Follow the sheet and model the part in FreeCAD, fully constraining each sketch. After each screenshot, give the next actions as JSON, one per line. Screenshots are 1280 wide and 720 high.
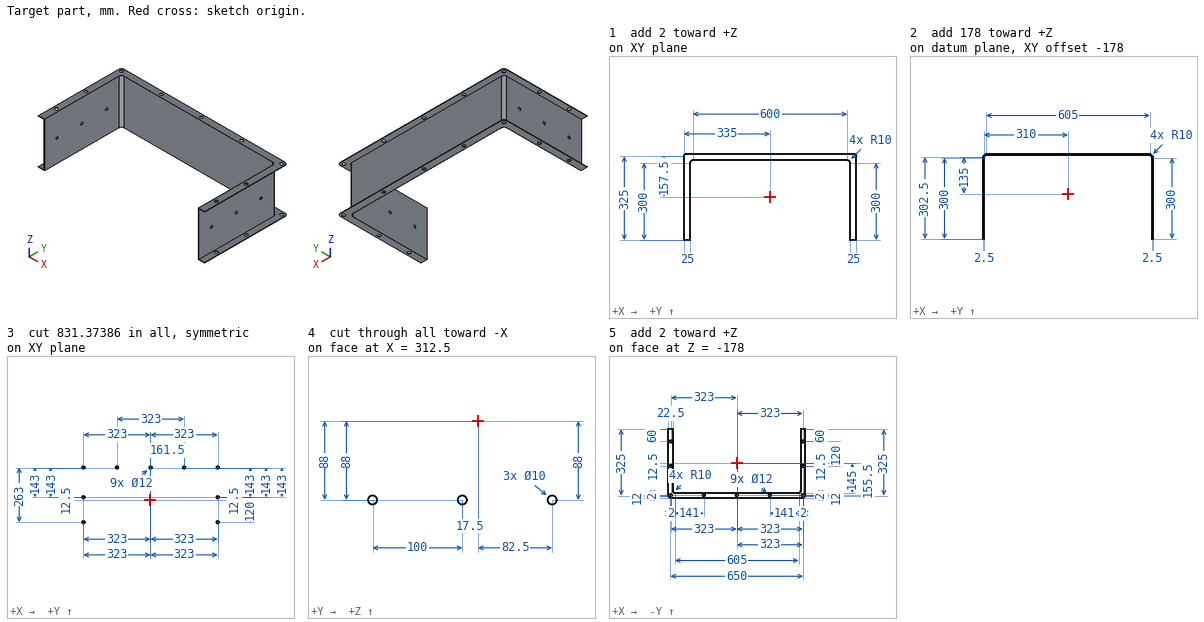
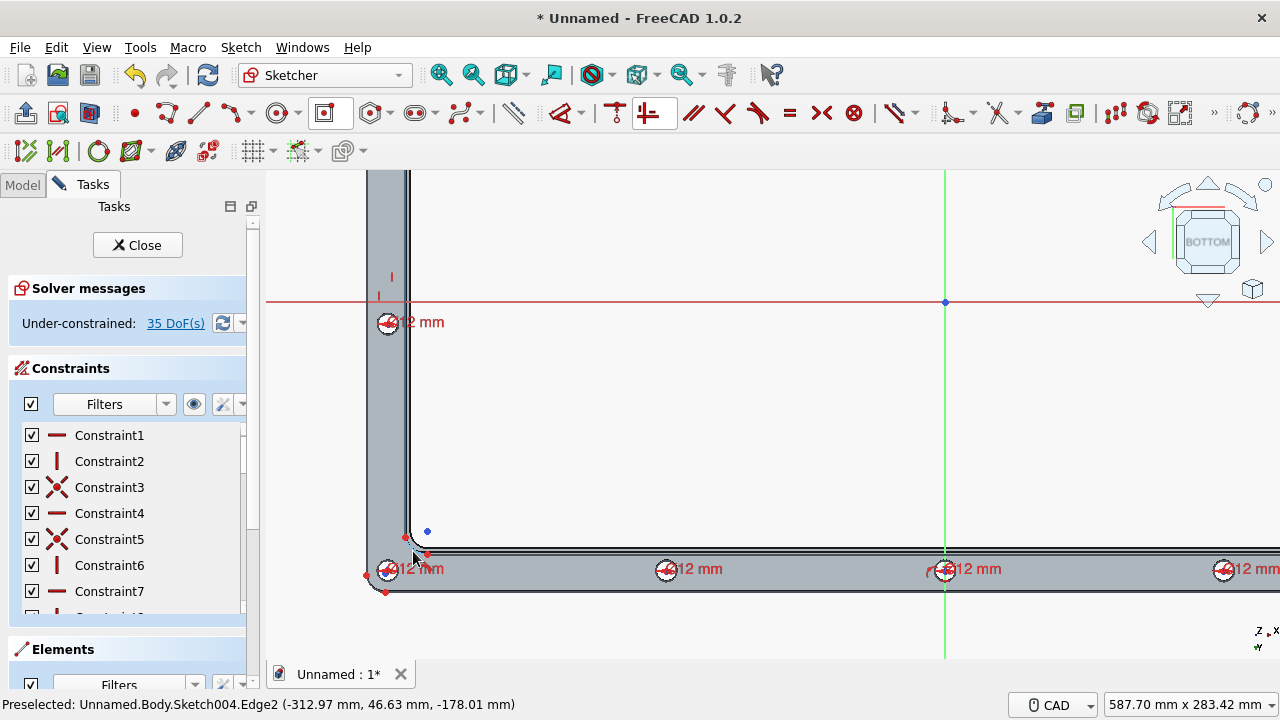
{"action": "left_click", "coordinate": [414, 550]}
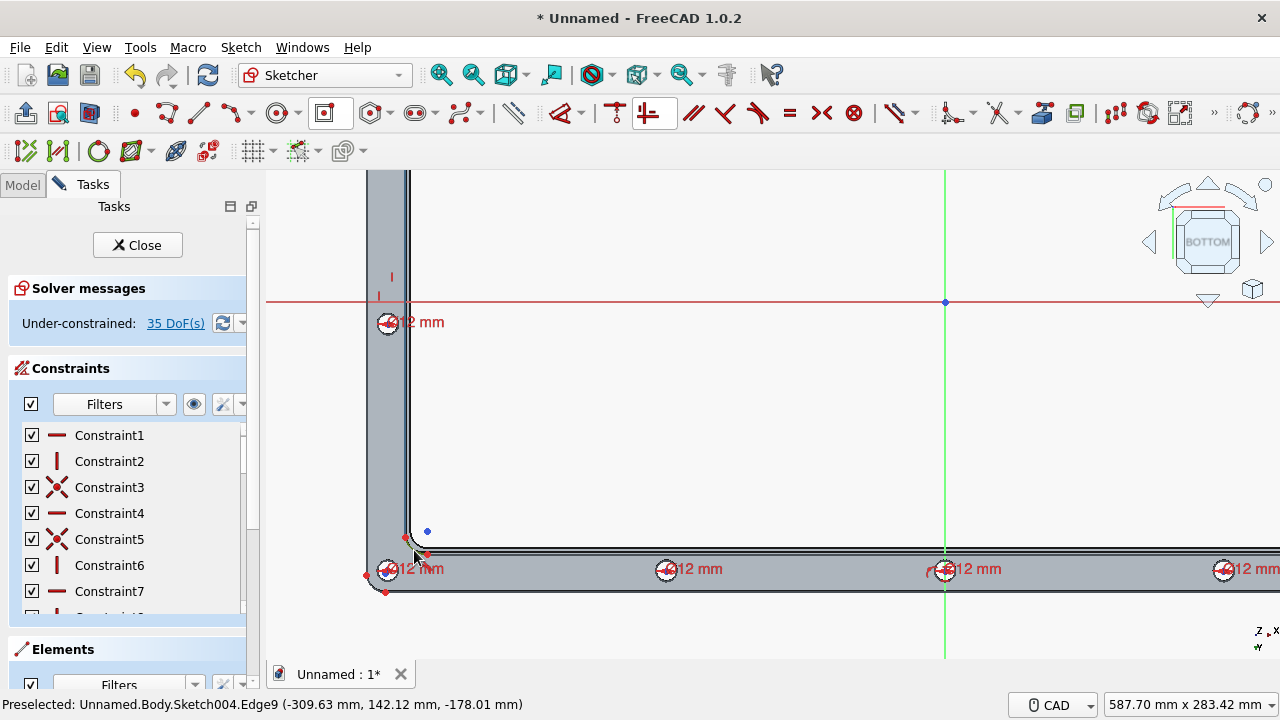
{"action": "left_click", "coordinate": [758, 114]}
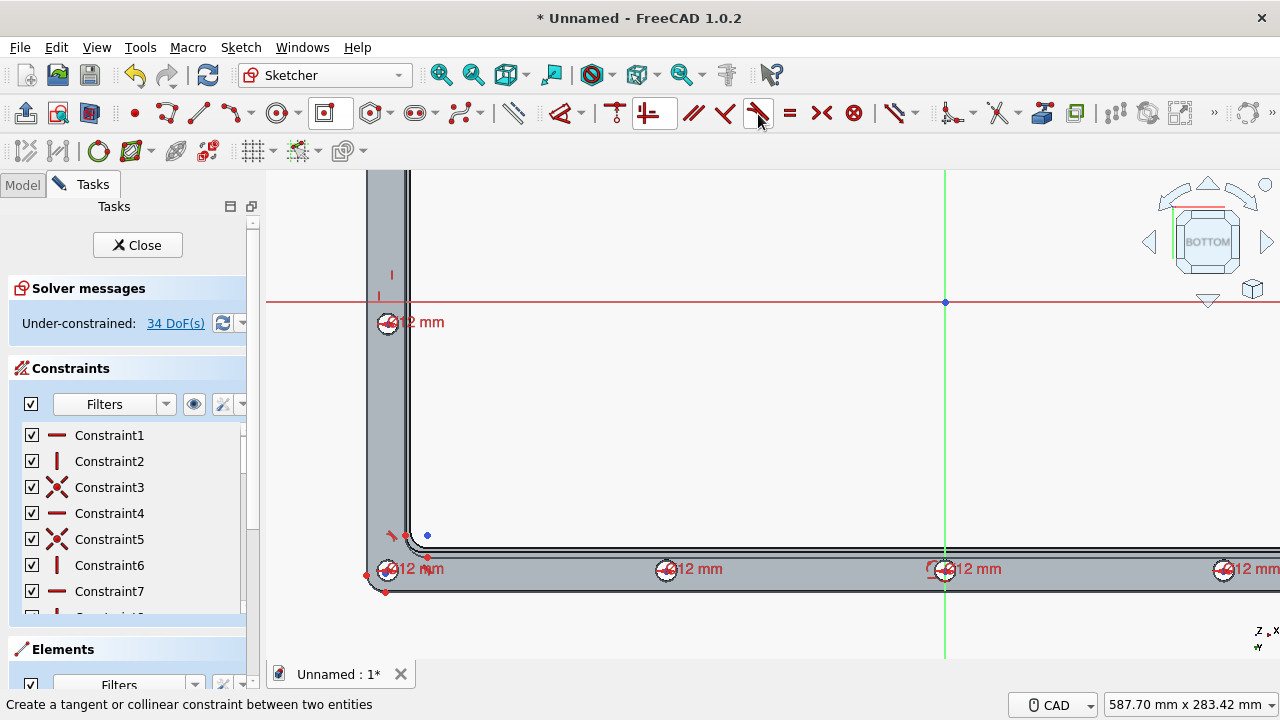
{"action": "left_click", "coordinate": [367, 408]}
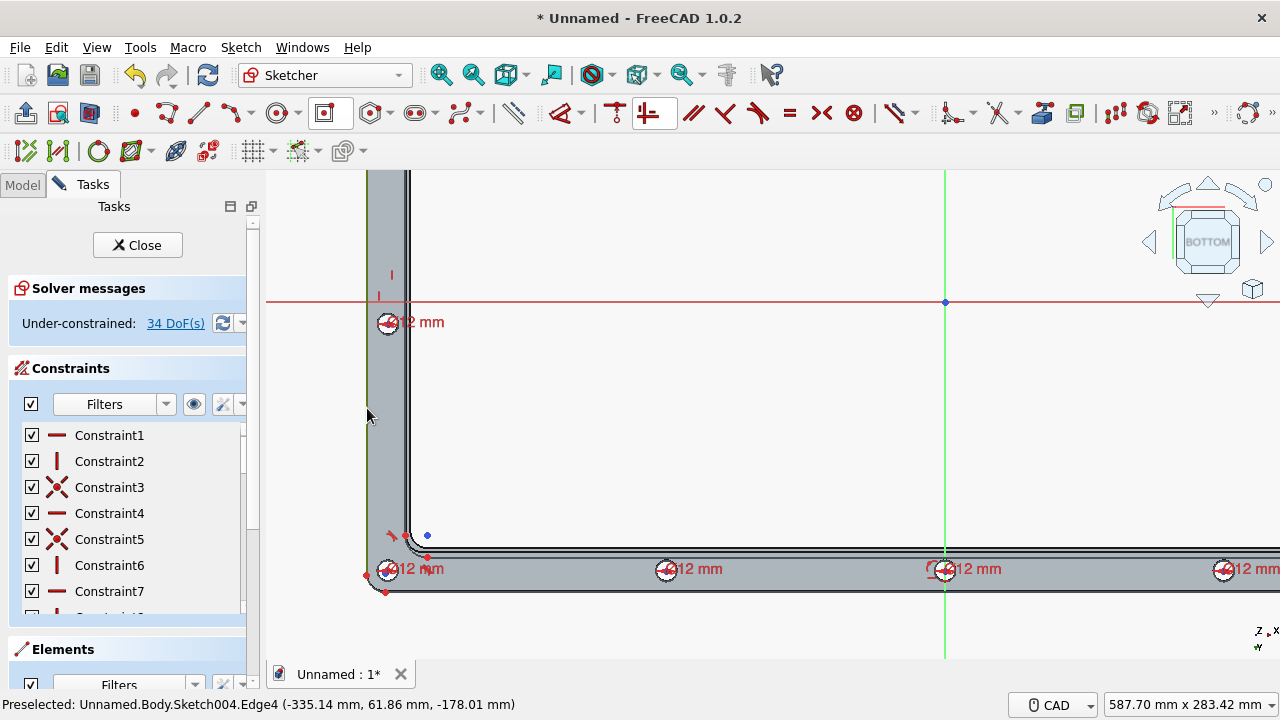
{"action": "left_click", "coordinate": [373, 587]}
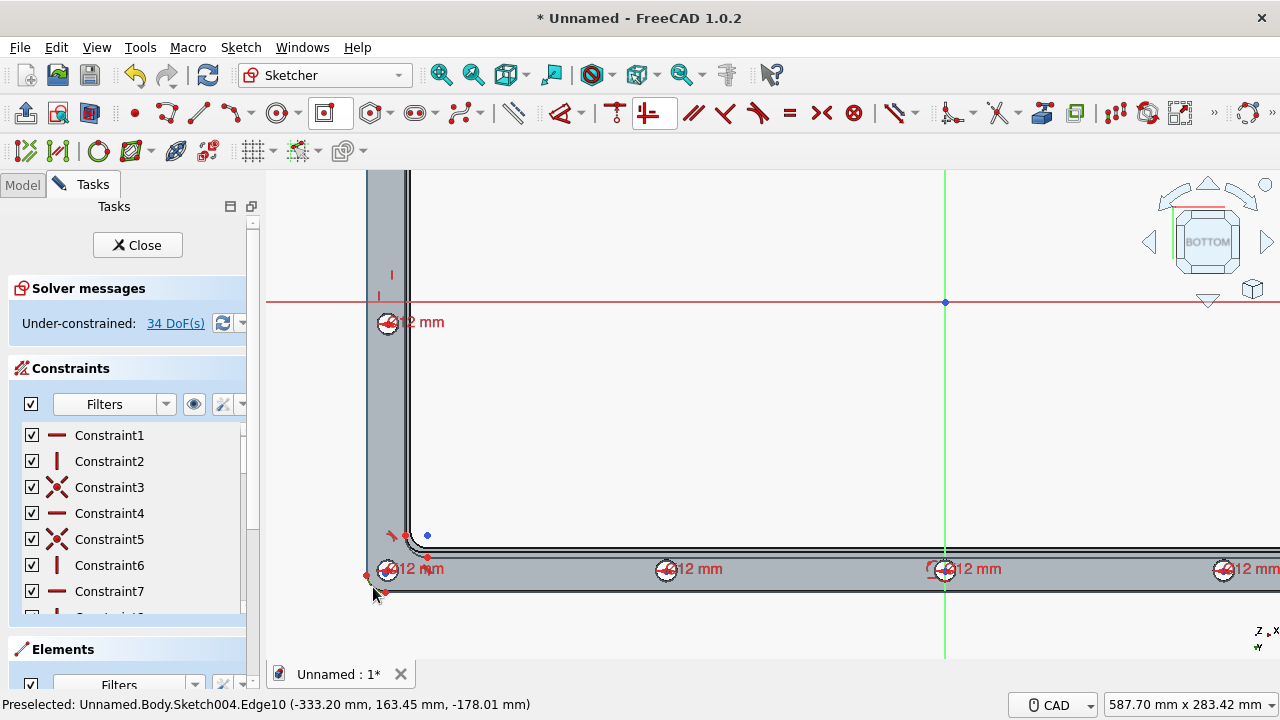
{"action": "key", "text": "t"}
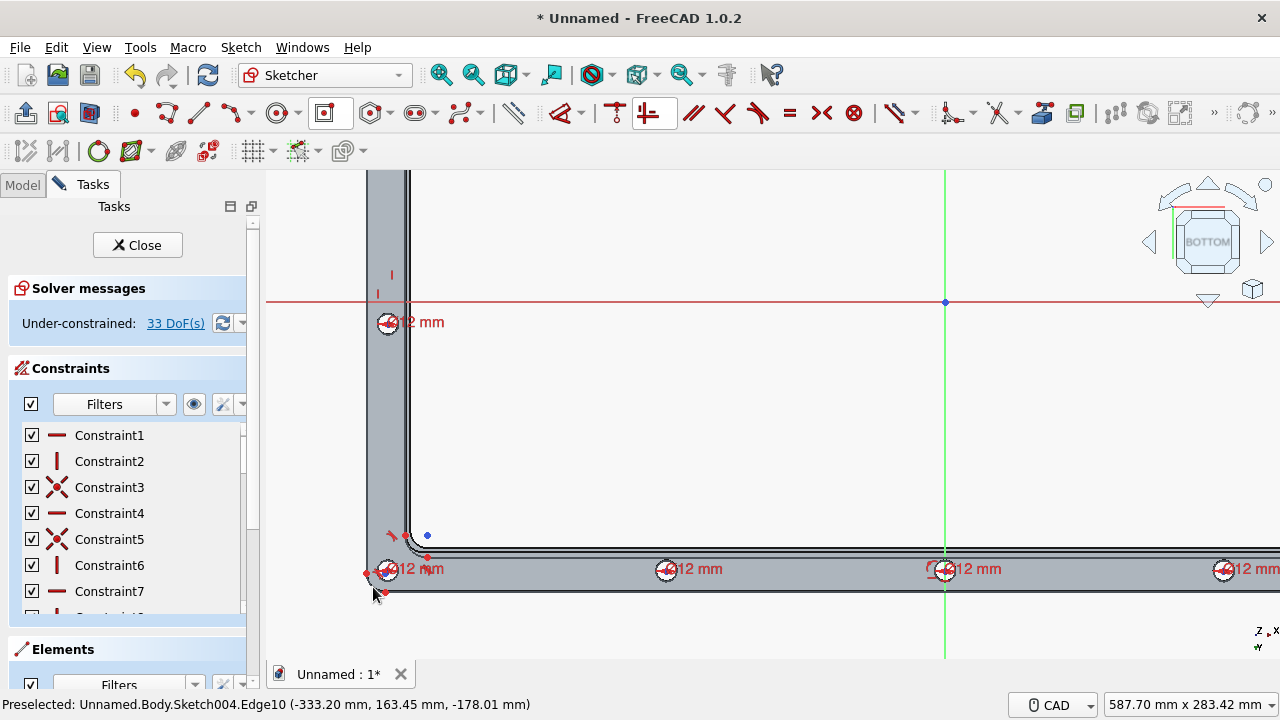
{"action": "left_click", "coordinate": [721, 592]}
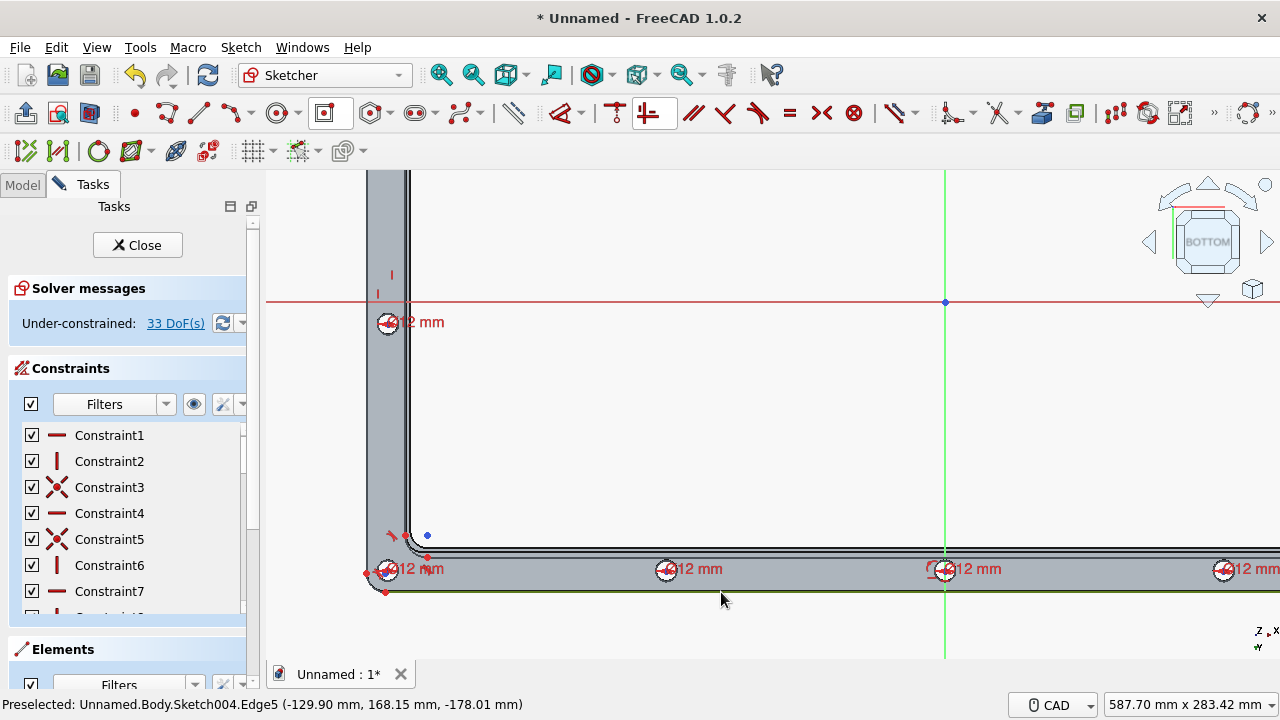
{"action": "left_click", "coordinate": [372, 586]}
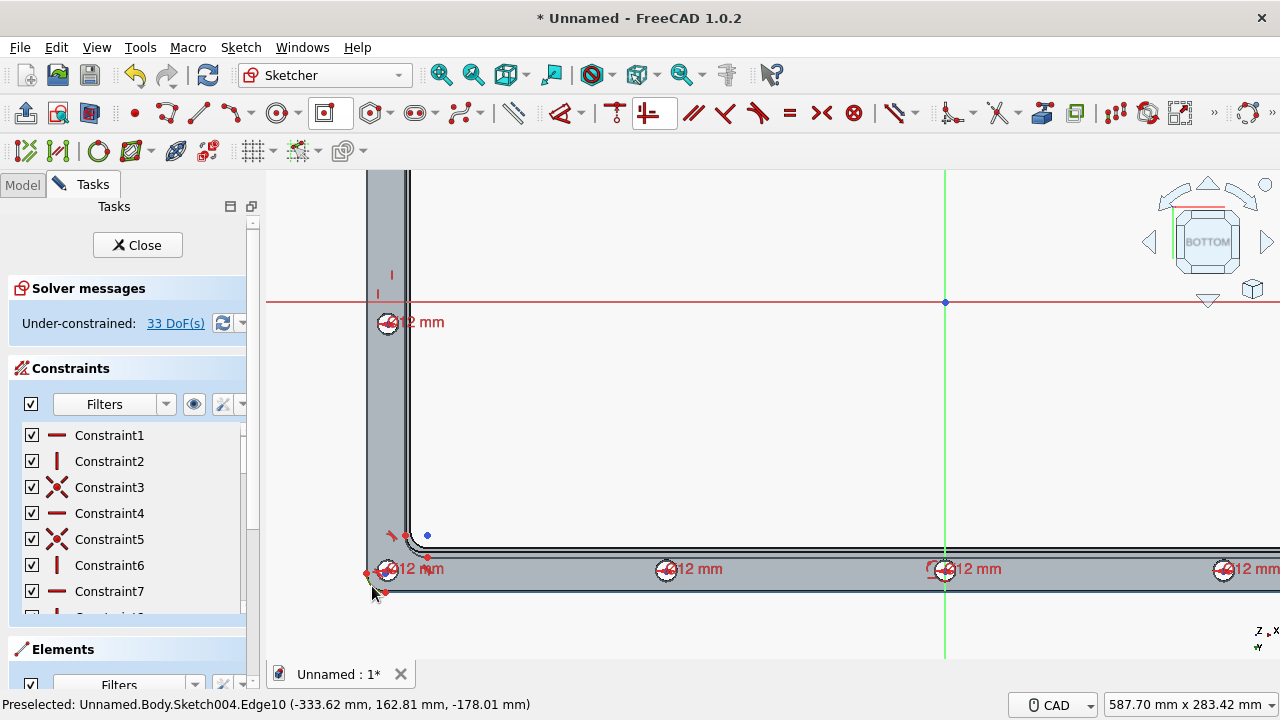
{"action": "left_click", "coordinate": [758, 114]}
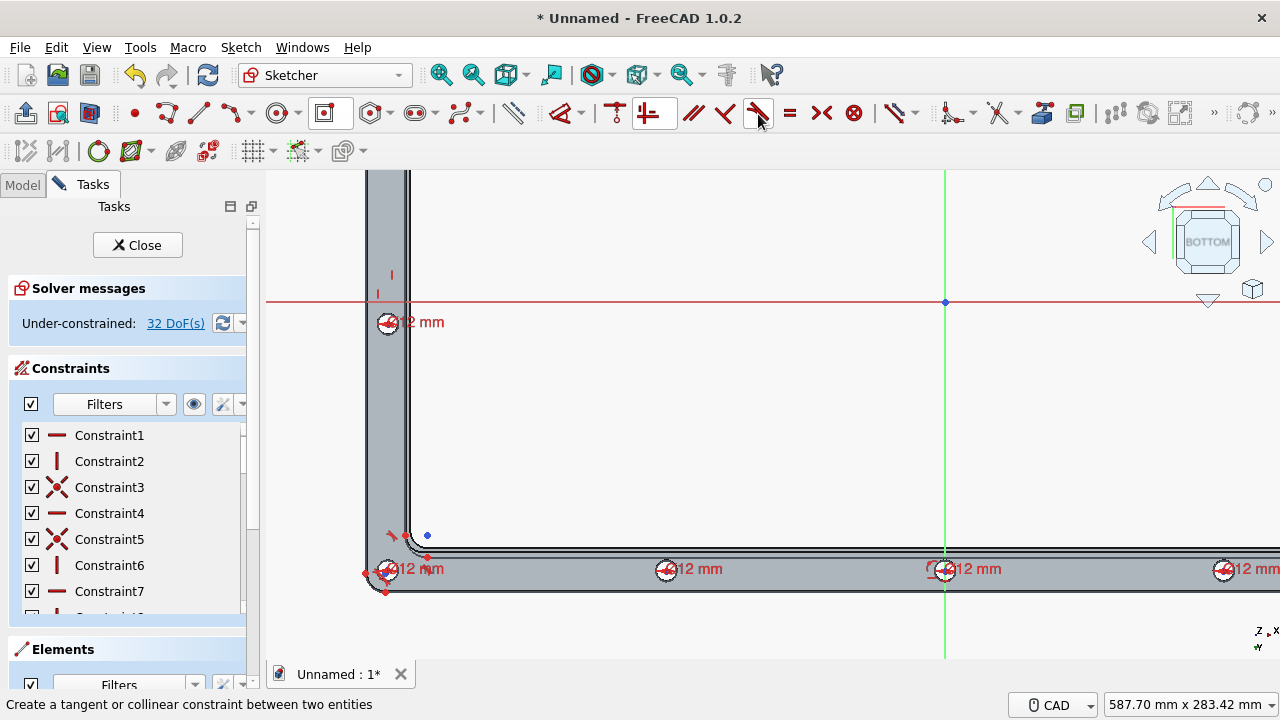
{"action": "left_click", "coordinate": [721, 592]}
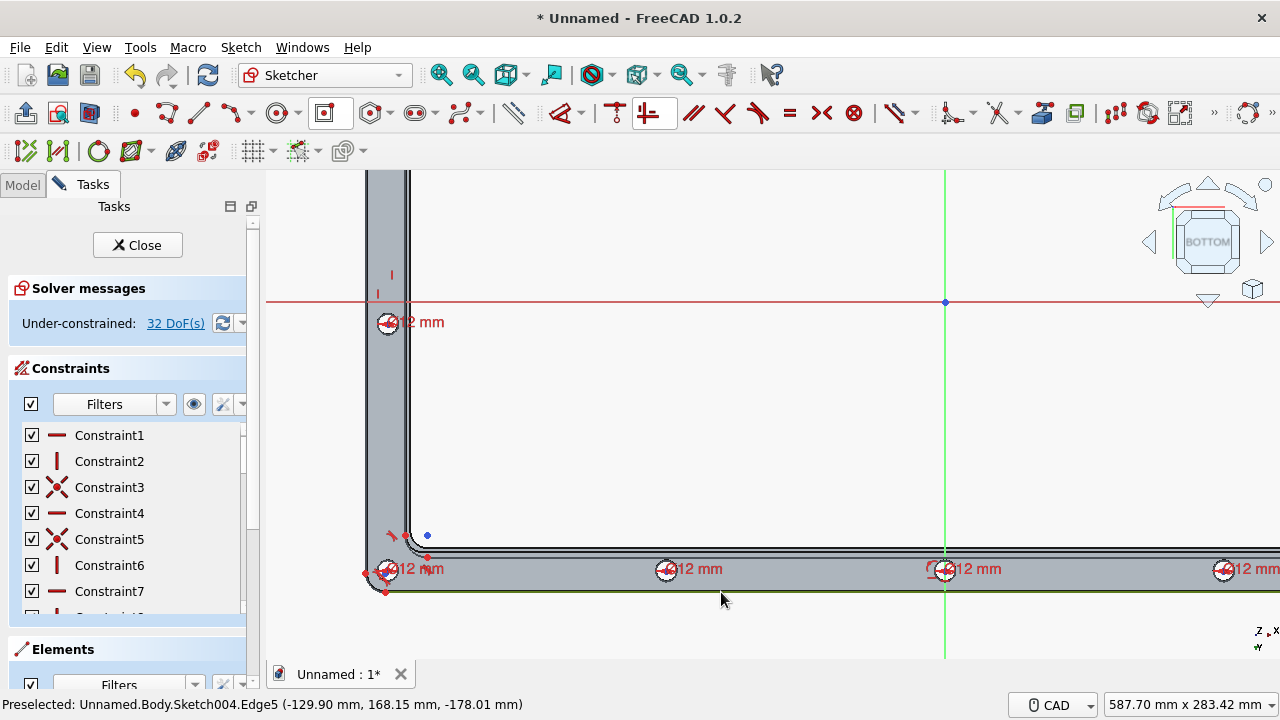
{"action": "scroll", "coordinate": [412, 551], "scroll_direction": "down", "scroll_amount": 3}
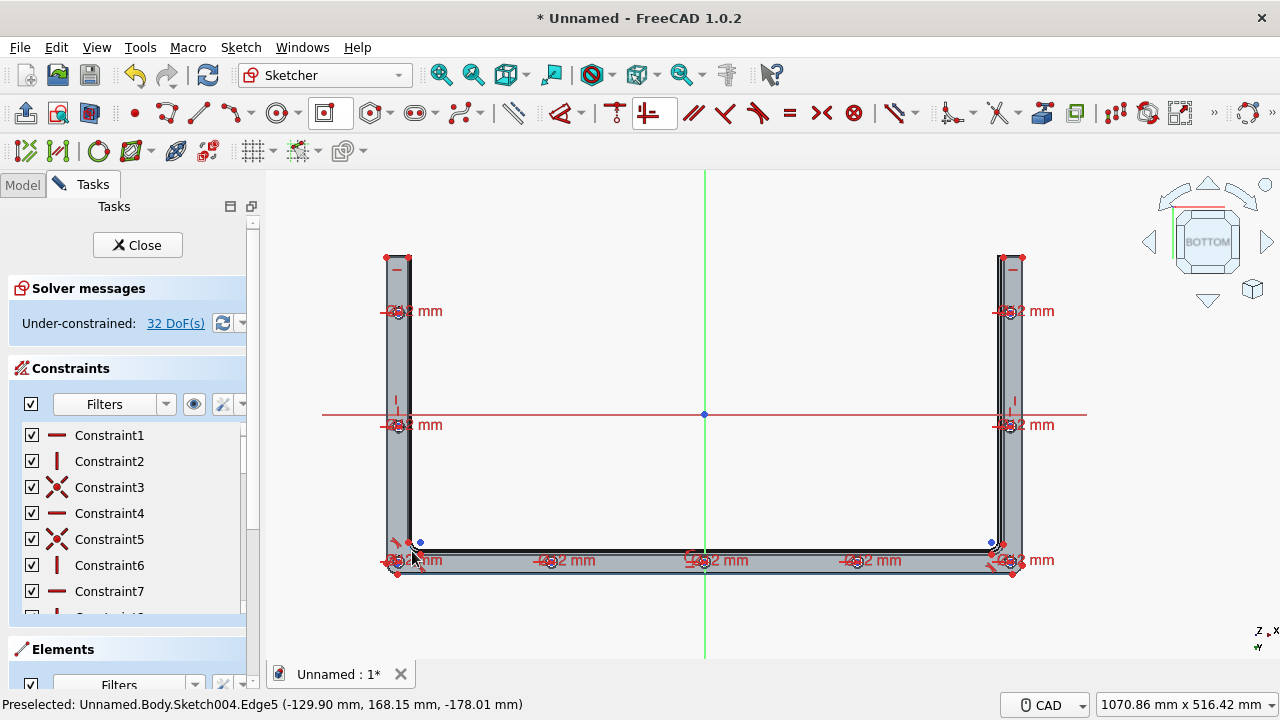
{"action": "scroll", "coordinate": [1019, 571], "scroll_direction": "up", "scroll_amount": 4}